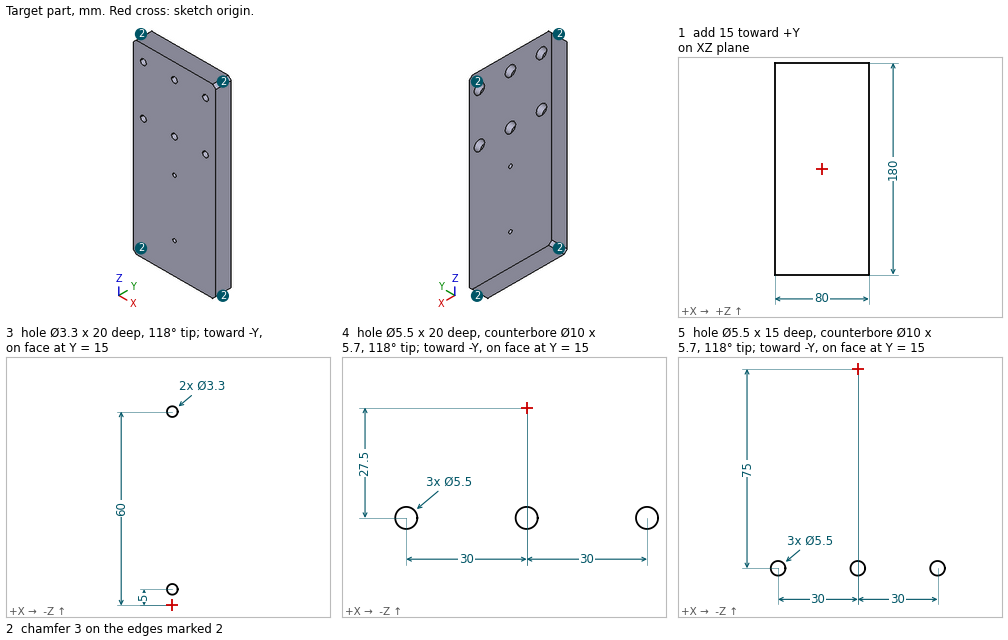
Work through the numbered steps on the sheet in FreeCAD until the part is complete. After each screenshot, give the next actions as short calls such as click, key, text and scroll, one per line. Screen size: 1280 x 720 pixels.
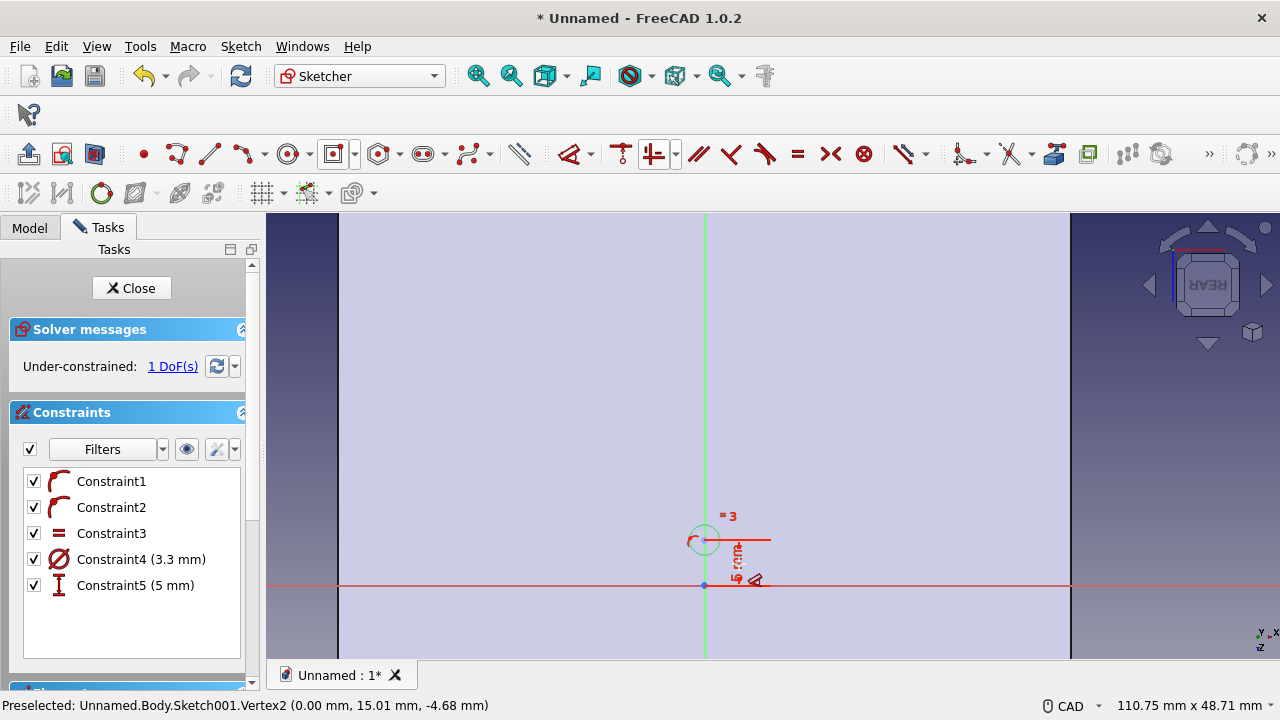
scroll(704, 544, down, 4)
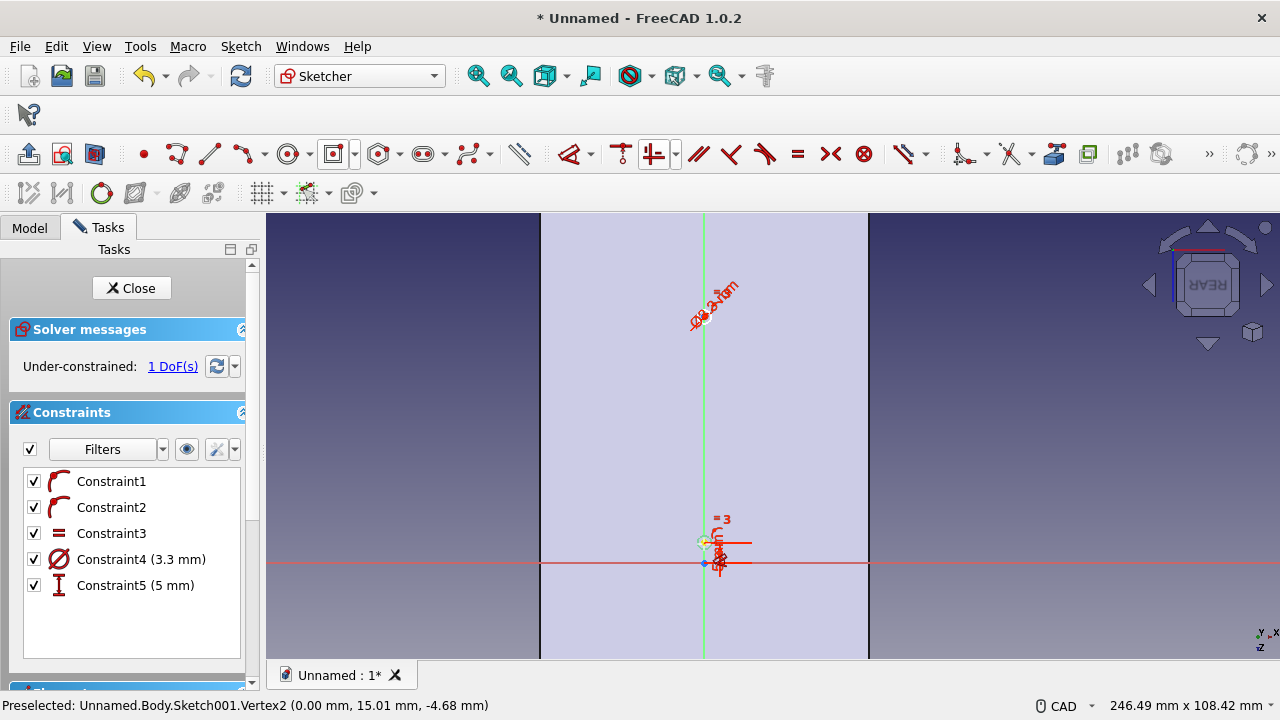
click(704, 317)
click(738, 440)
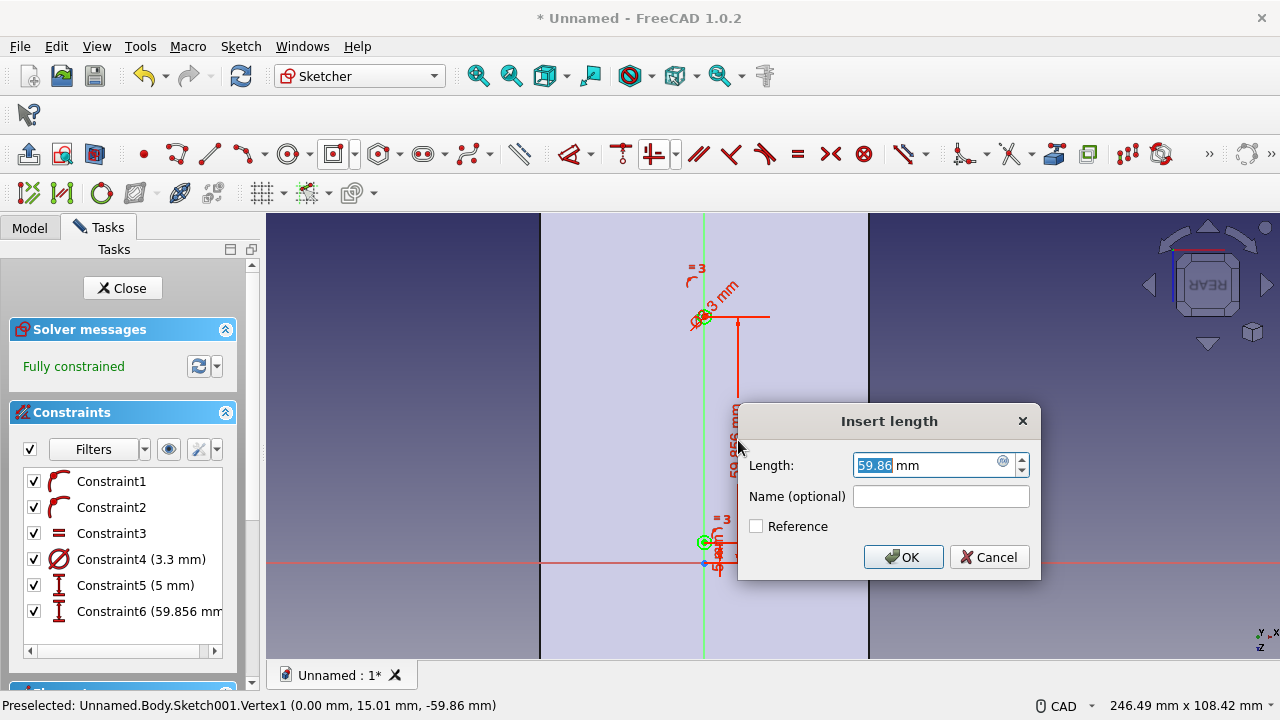
text(60)
key(Return)
key(Escape)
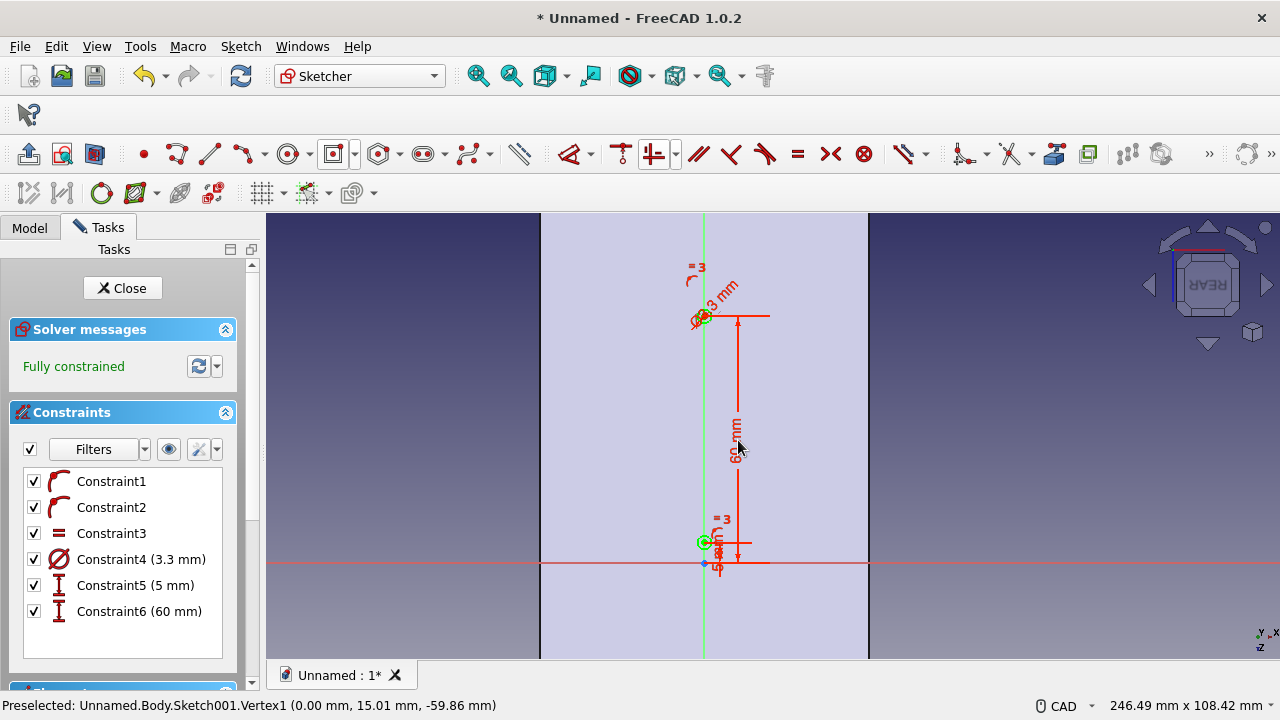
click(123, 288)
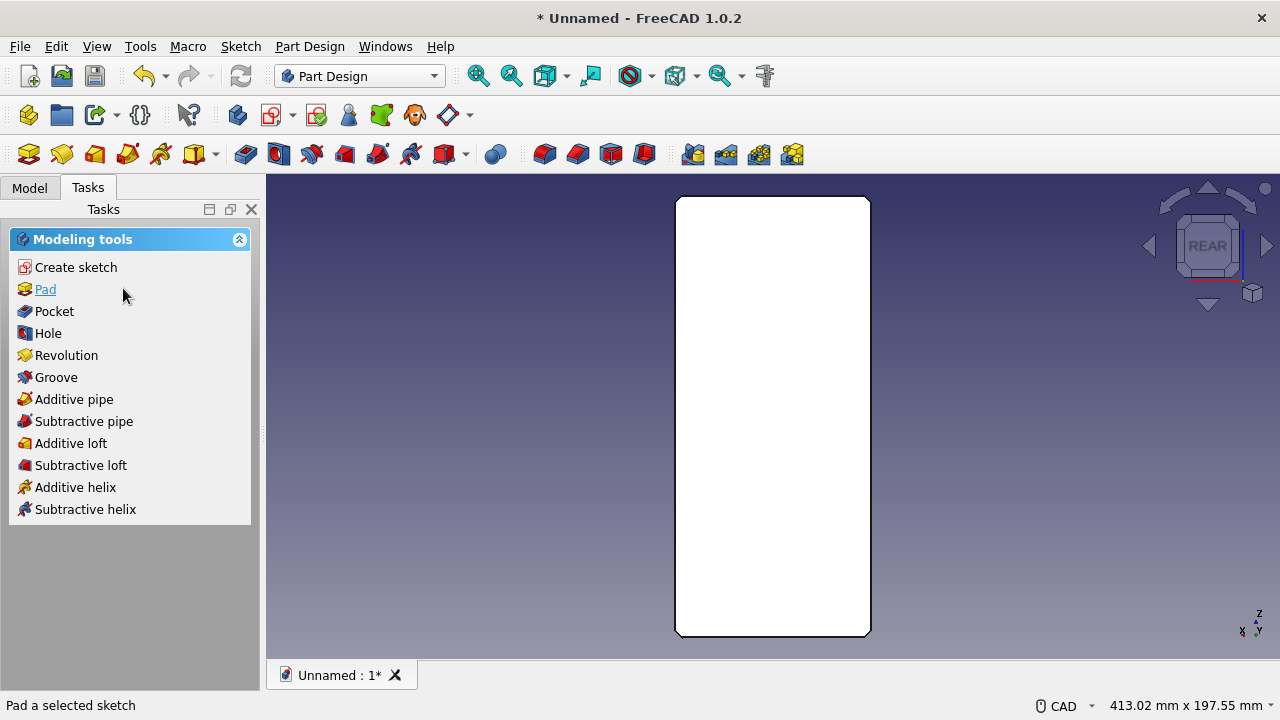
click(279, 154)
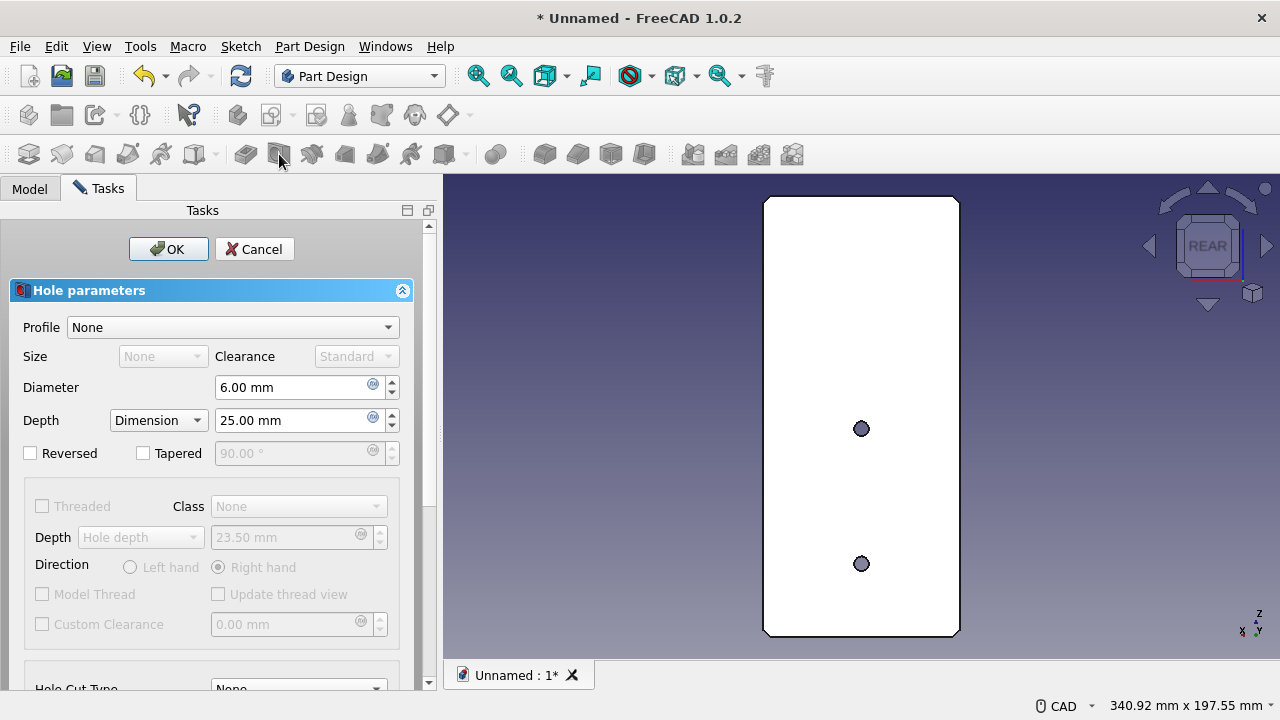
triple_click(300, 388)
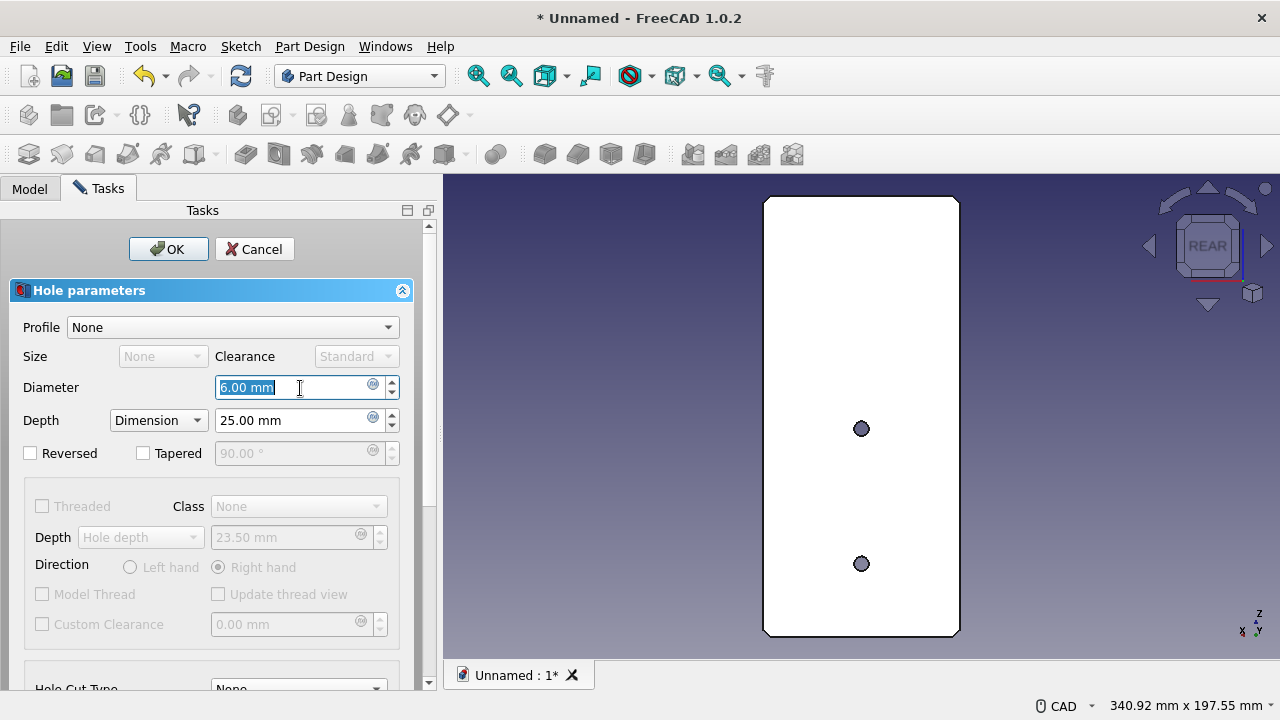
text(3.3)
key(Tab)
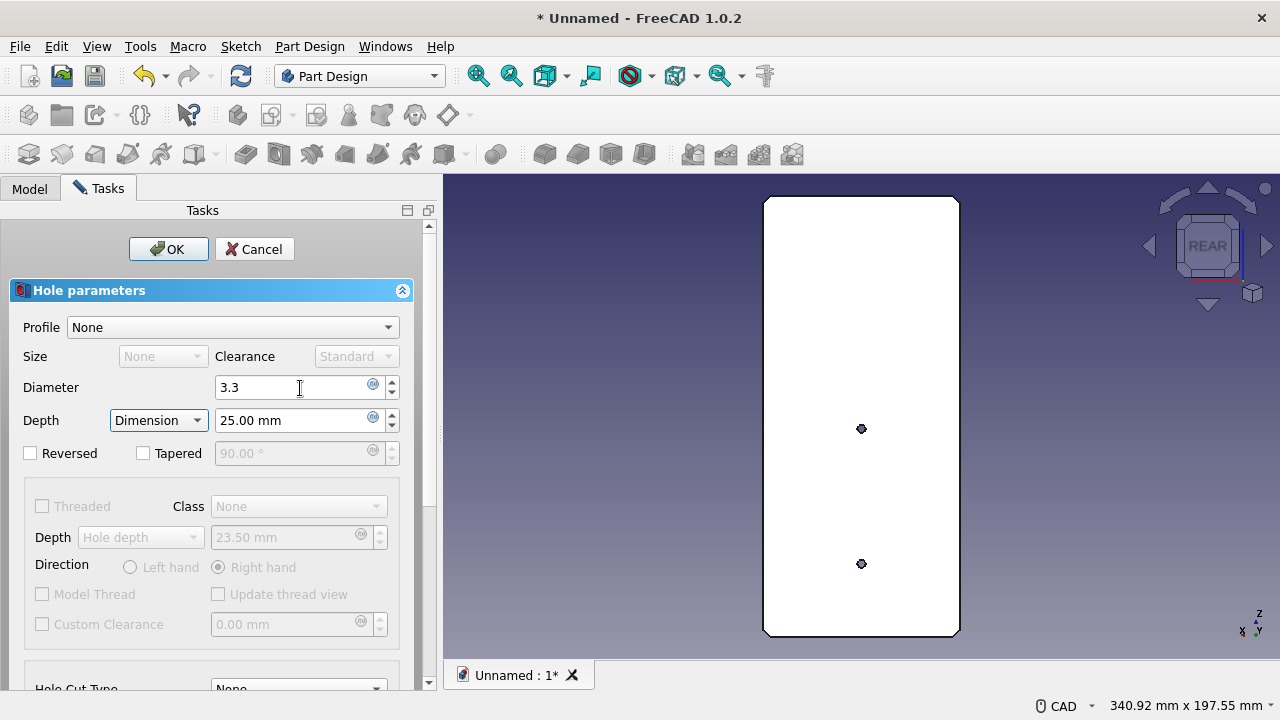
triple_click(300, 420)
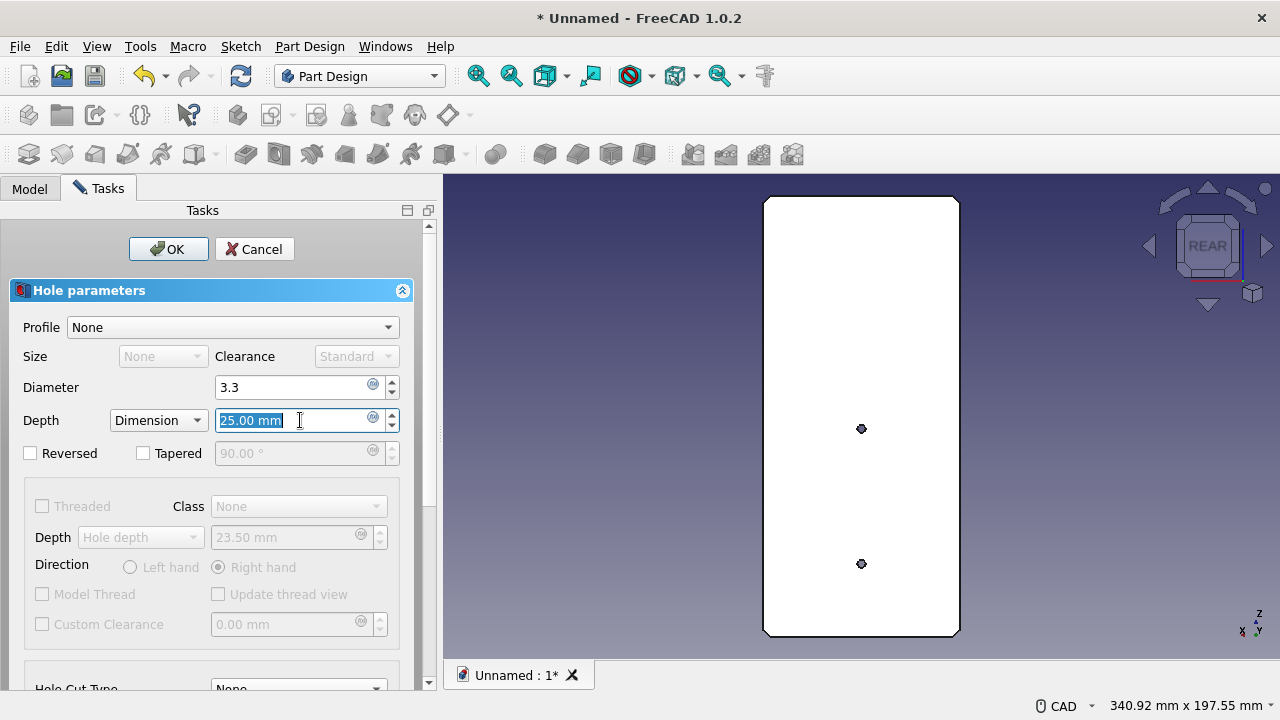
text(20)
key(Tab)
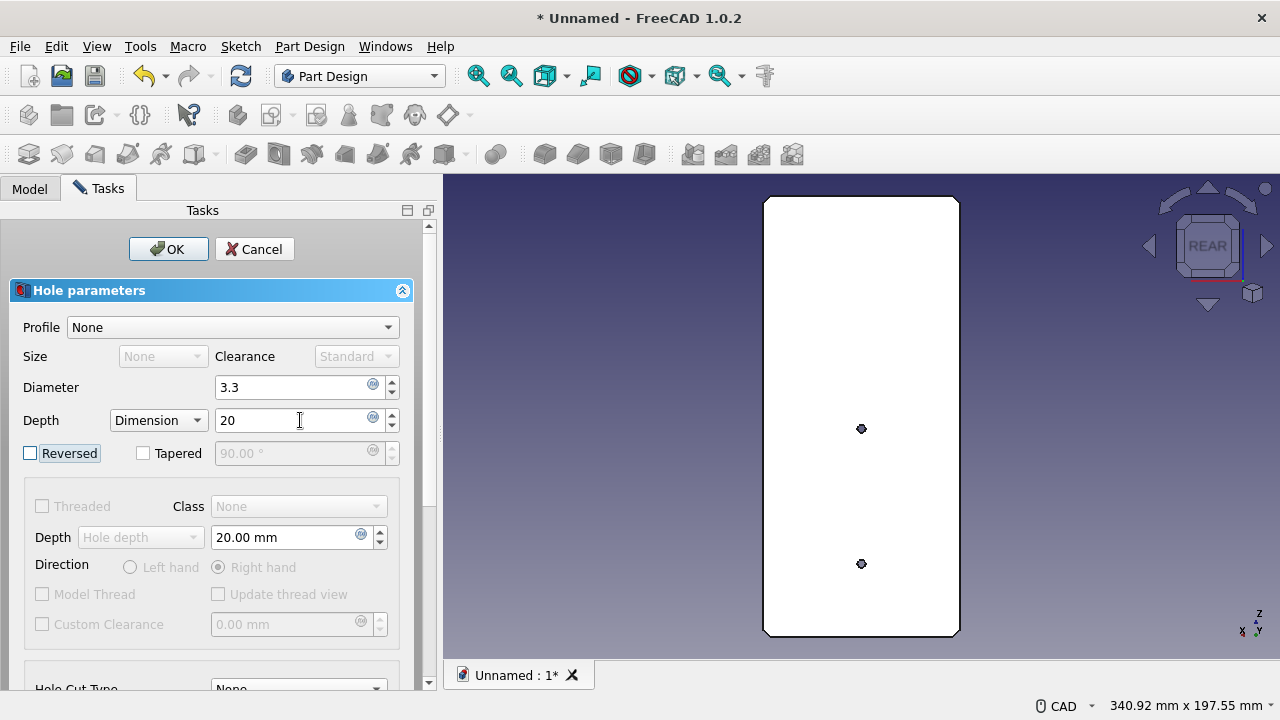
click(169, 249)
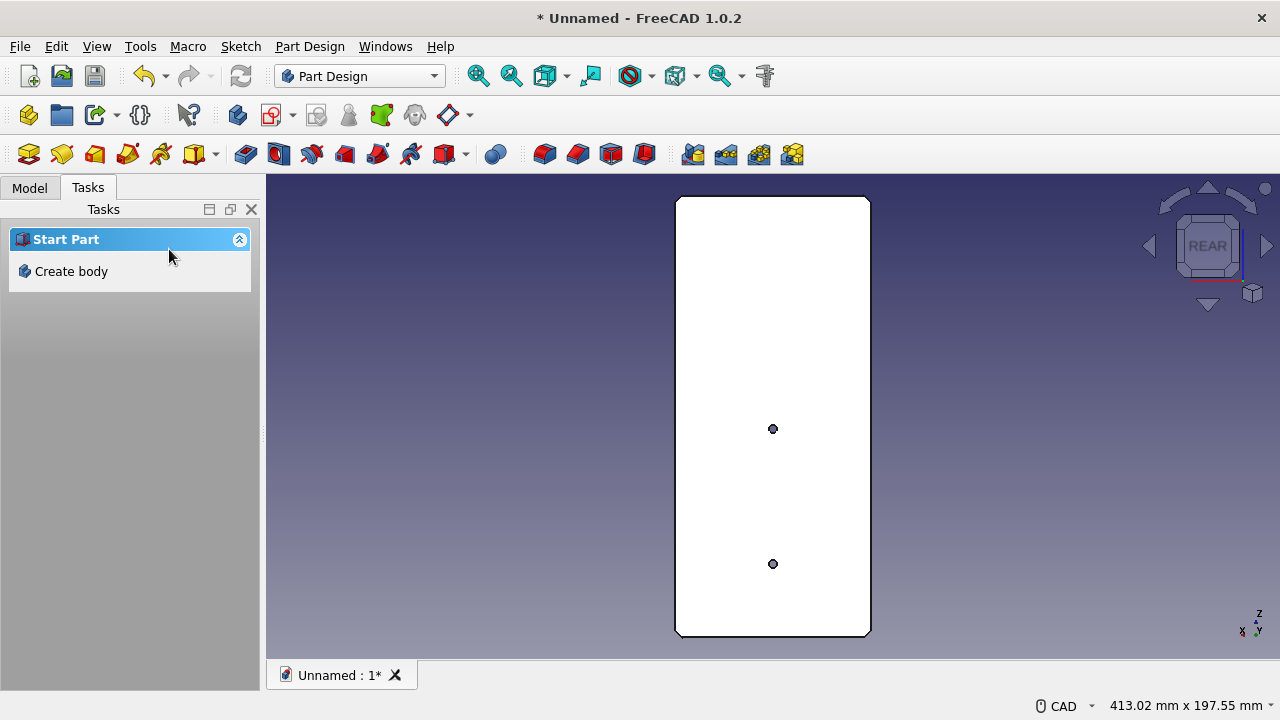
click(773, 289)